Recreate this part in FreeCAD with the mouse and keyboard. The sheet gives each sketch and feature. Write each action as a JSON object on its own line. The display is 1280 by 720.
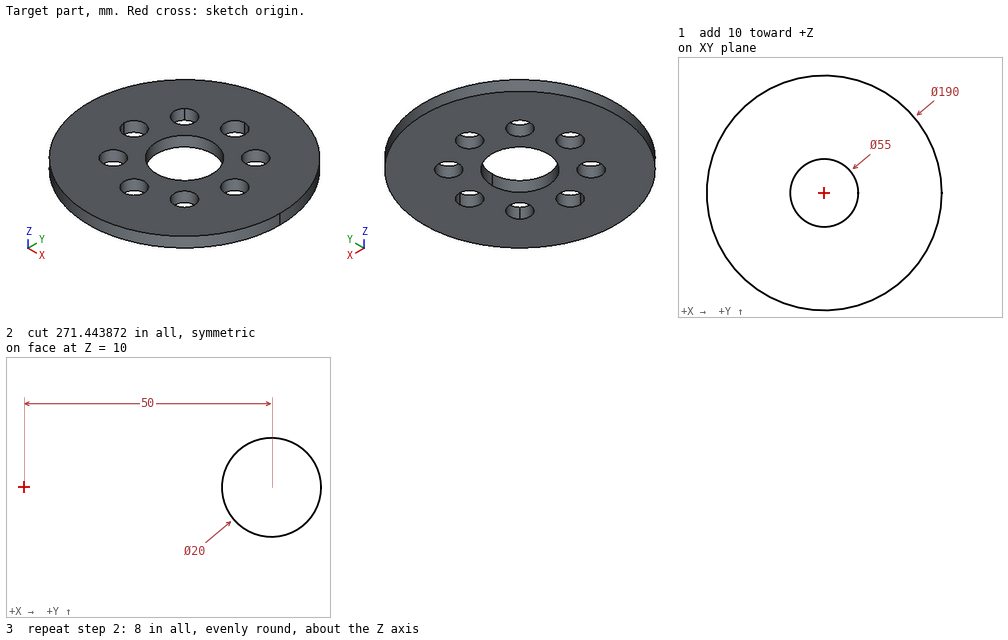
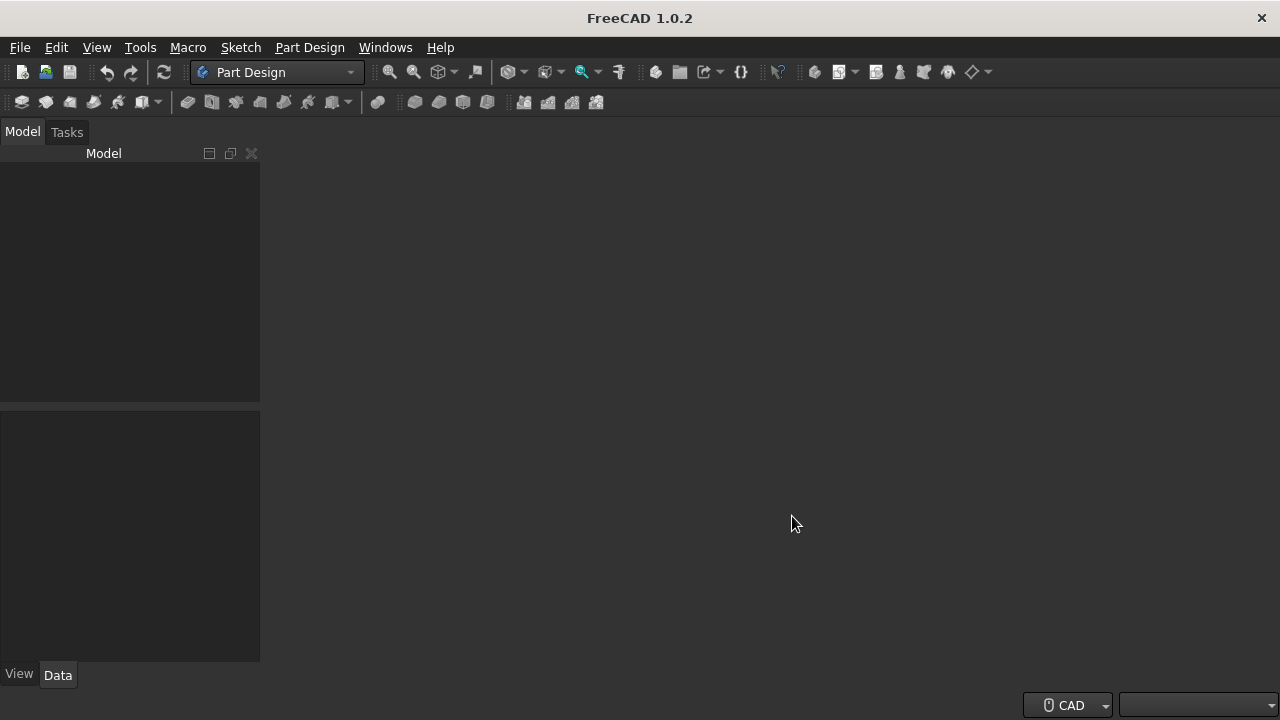
{"action": "left_click", "coordinate": [22, 72]}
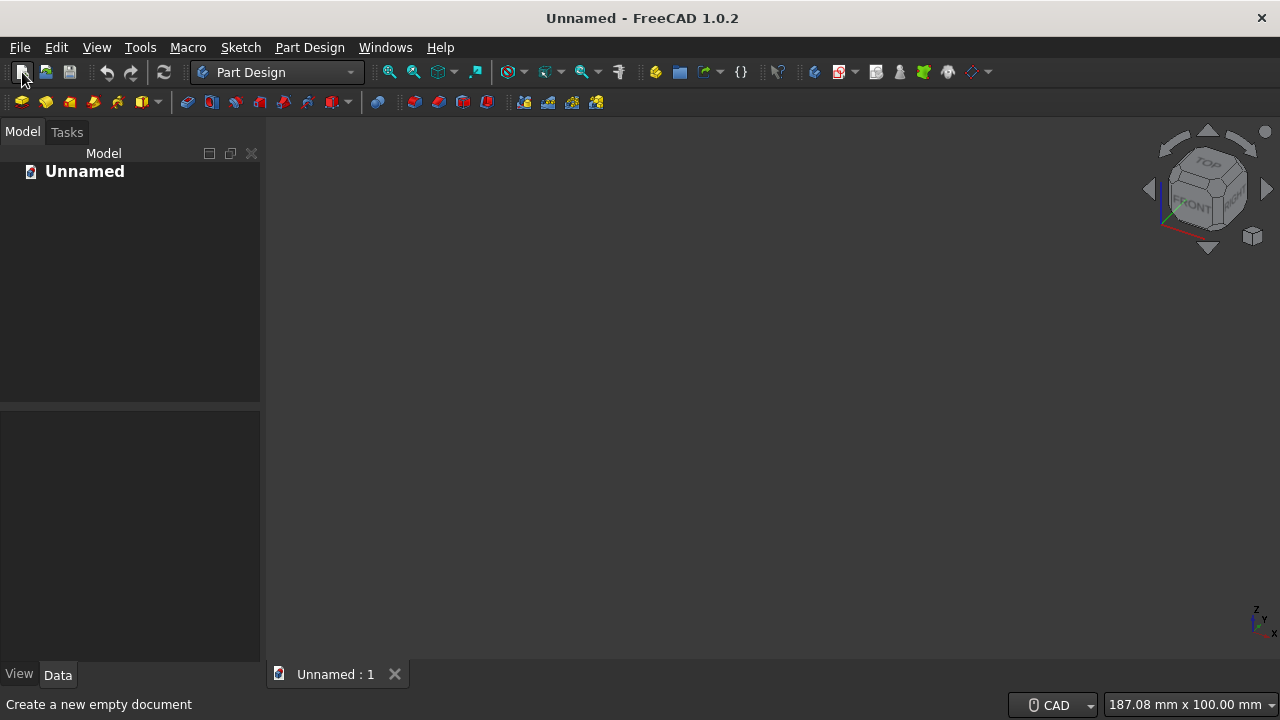
{"action": "left_click", "coordinate": [840, 72]}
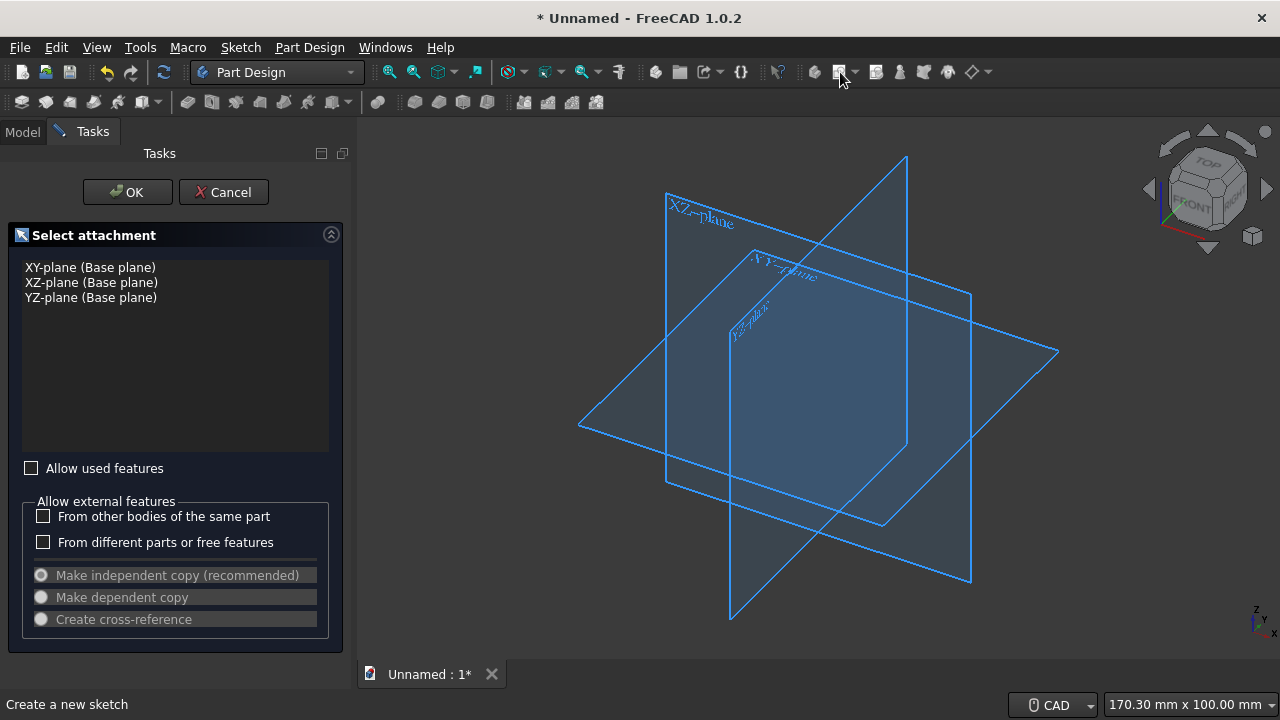
{"action": "left_click", "coordinate": [82, 268]}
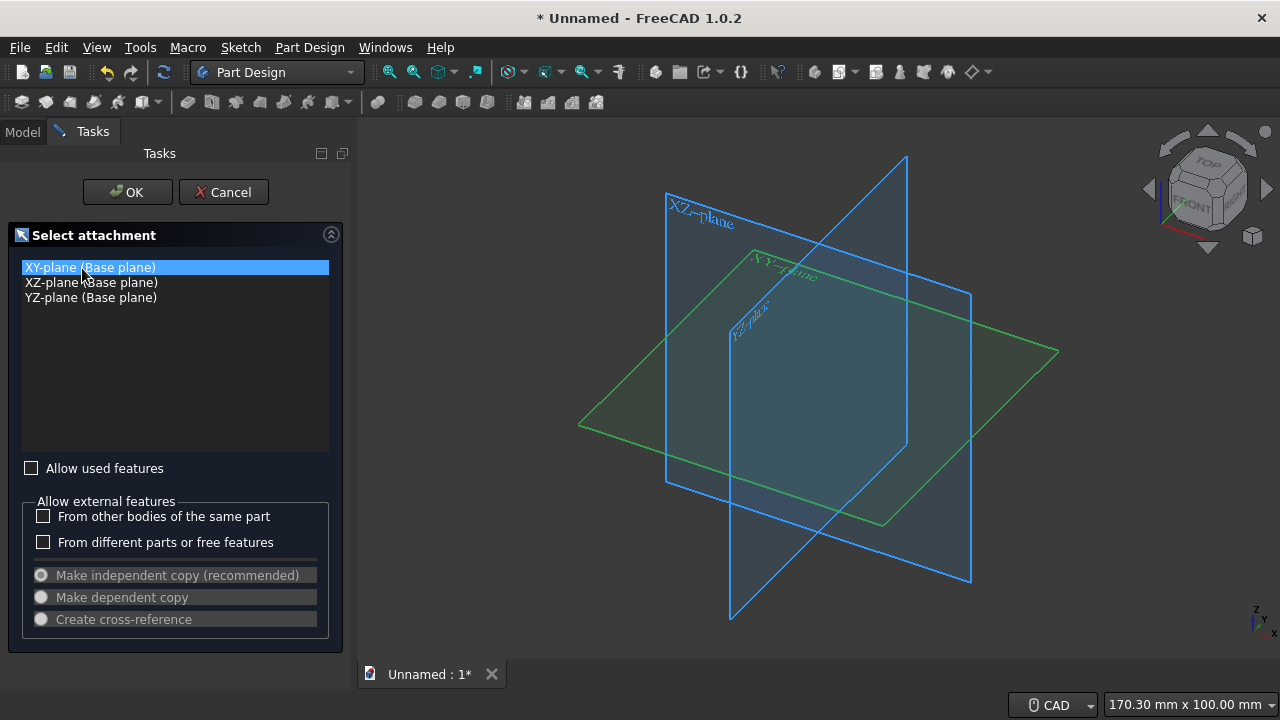
{"action": "left_click", "coordinate": [128, 192]}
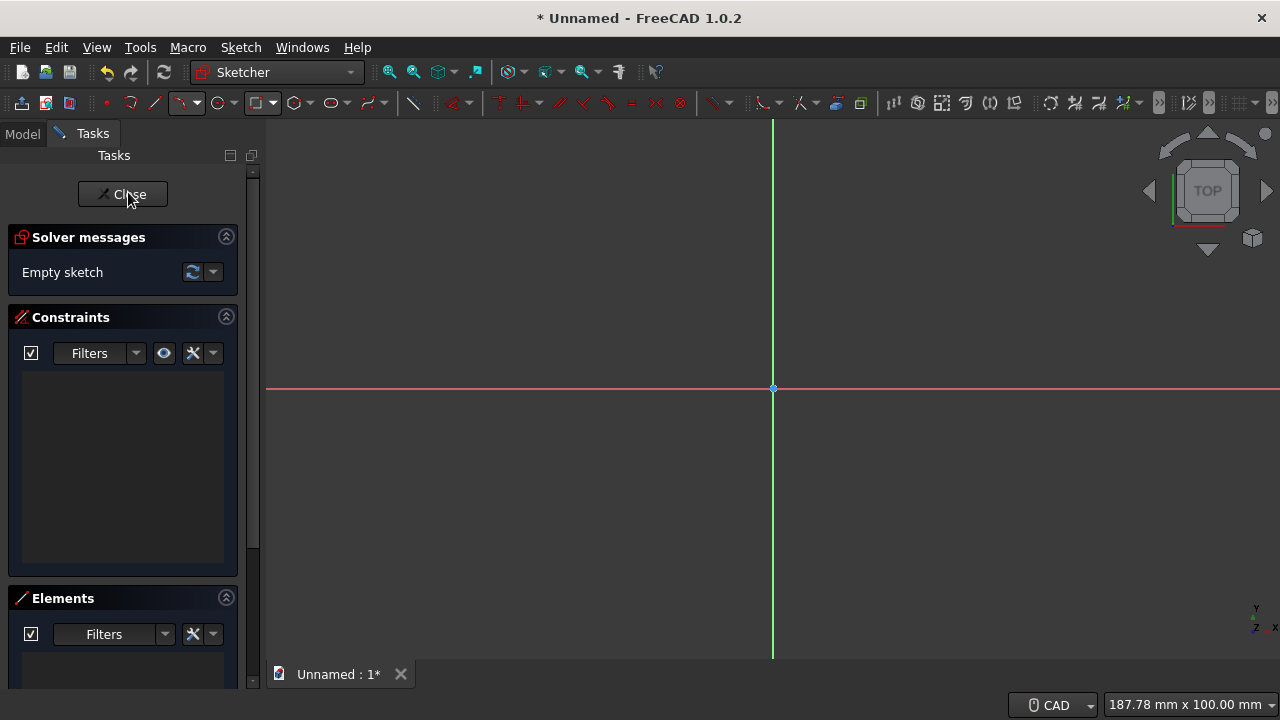
{"action": "scroll", "coordinate": [665, 389], "scroll_direction": "down", "scroll_amount": 5}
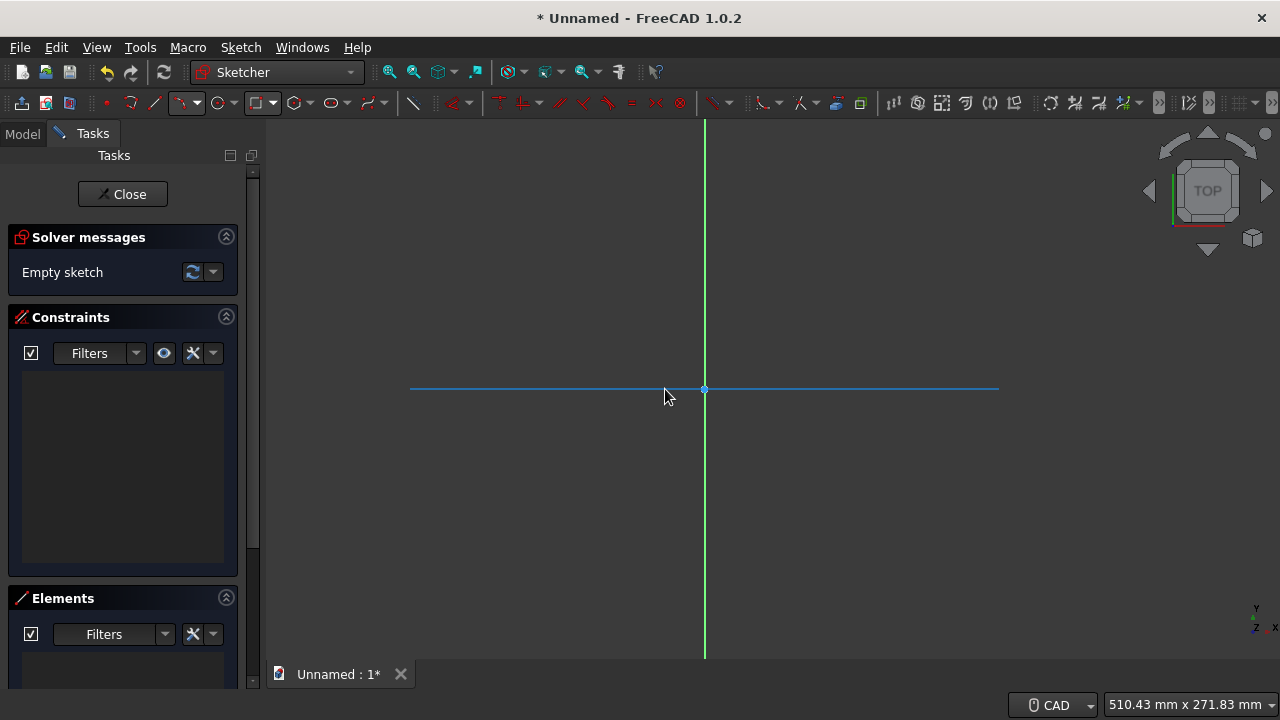
{"action": "left_click", "coordinate": [218, 104]}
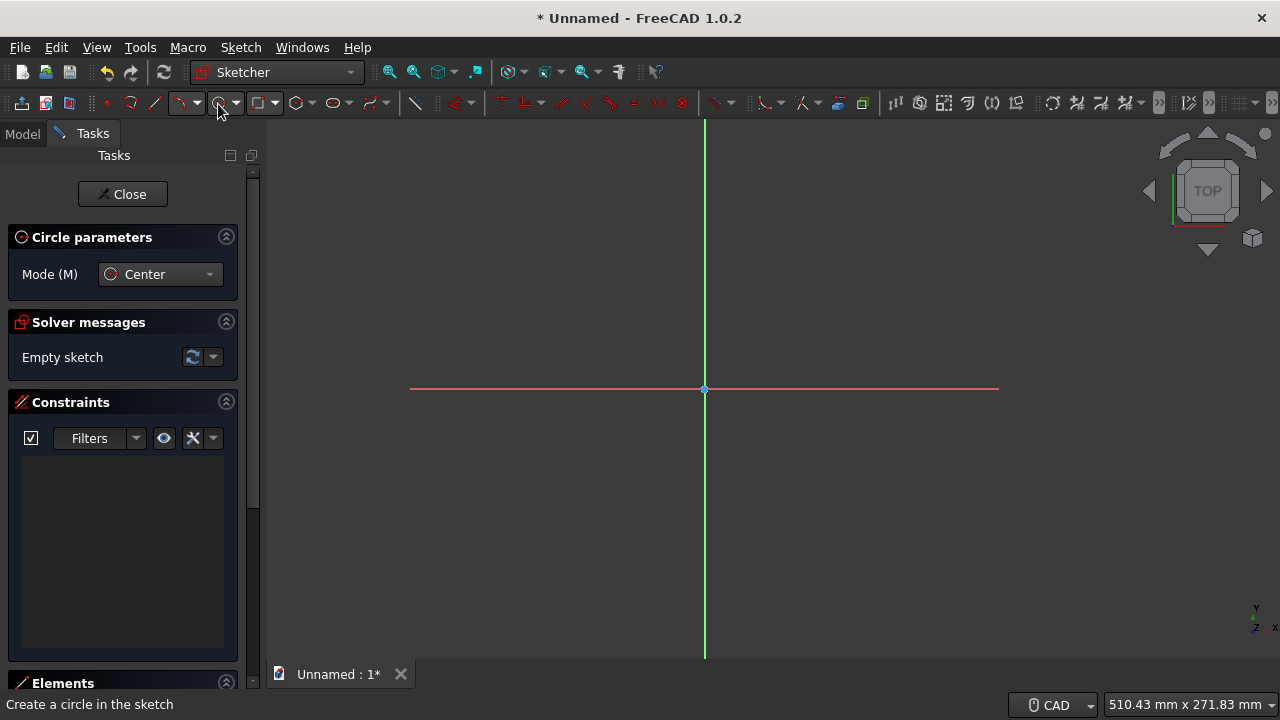
{"action": "left_click", "coordinate": [705, 389]}
{"action": "mouse_move", "coordinate": [838, 256]}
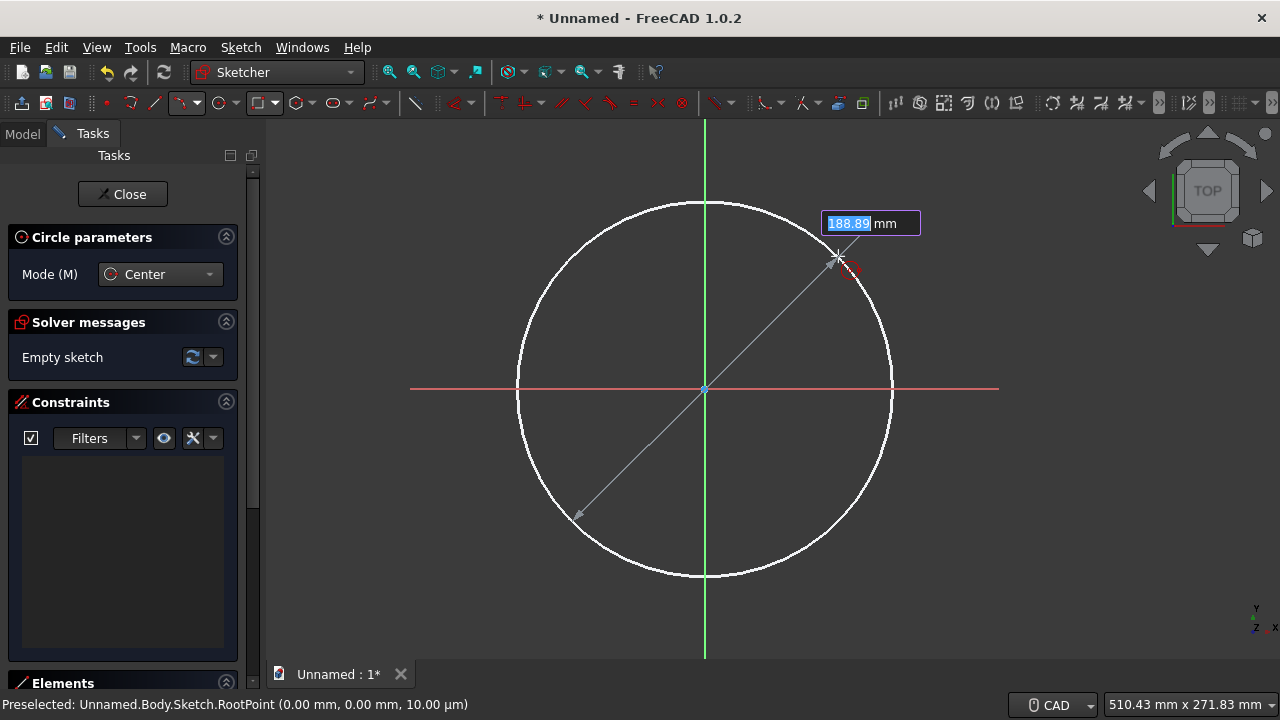
{"action": "type", "text": "190"}
{"action": "key", "text": "Return"}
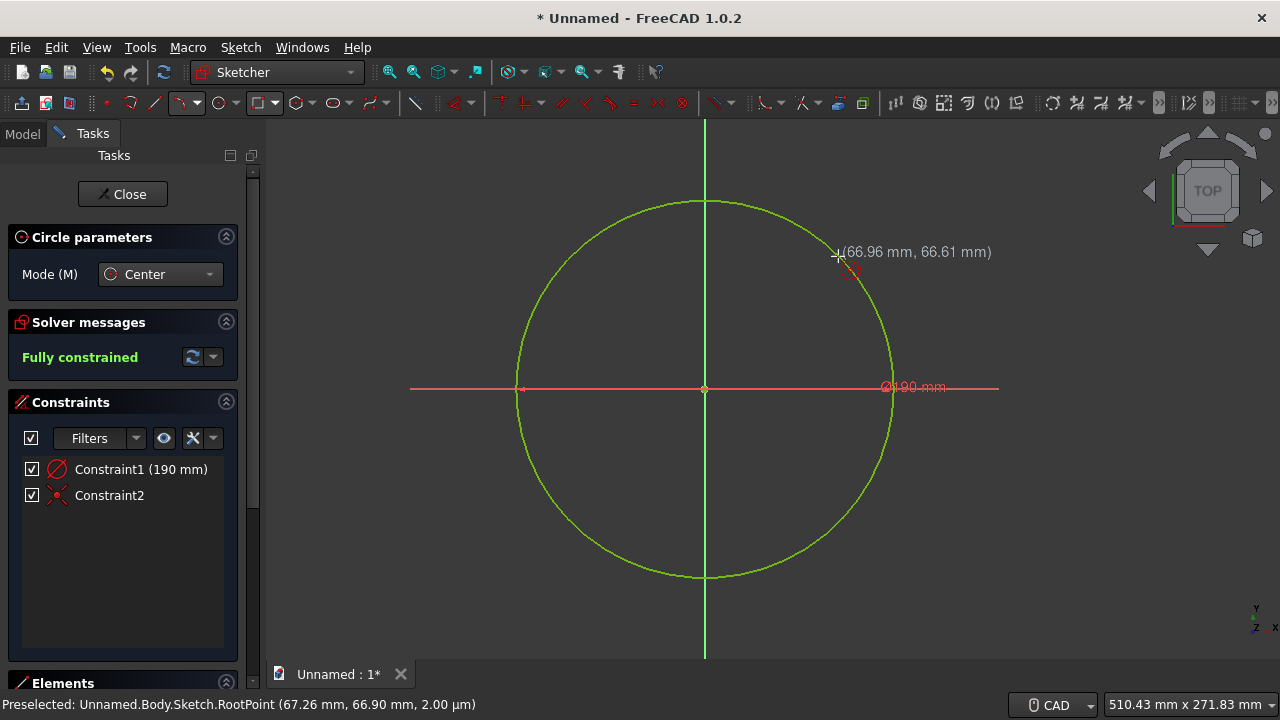
{"action": "left_click", "coordinate": [705, 389]}
{"action": "mouse_move", "coordinate": [744, 351]}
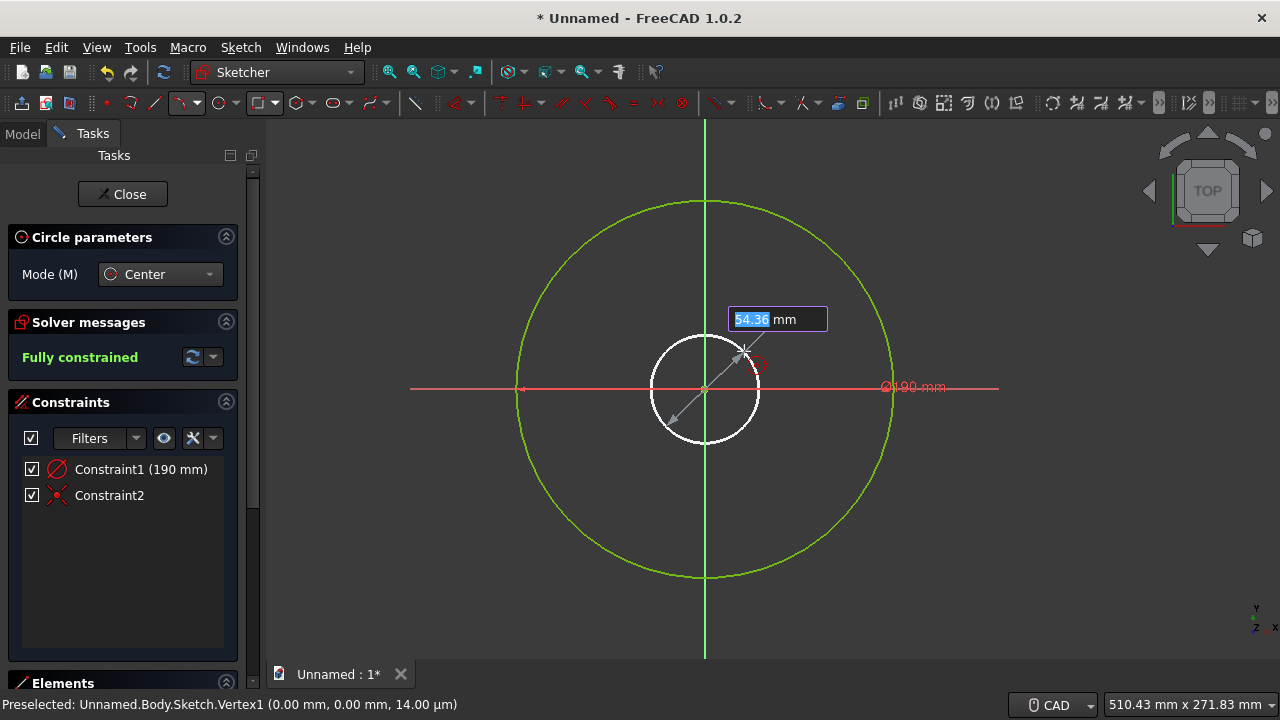
{"action": "type", "text": "55"}
{"action": "key", "text": "Return"}
{"action": "key", "text": "Escape"}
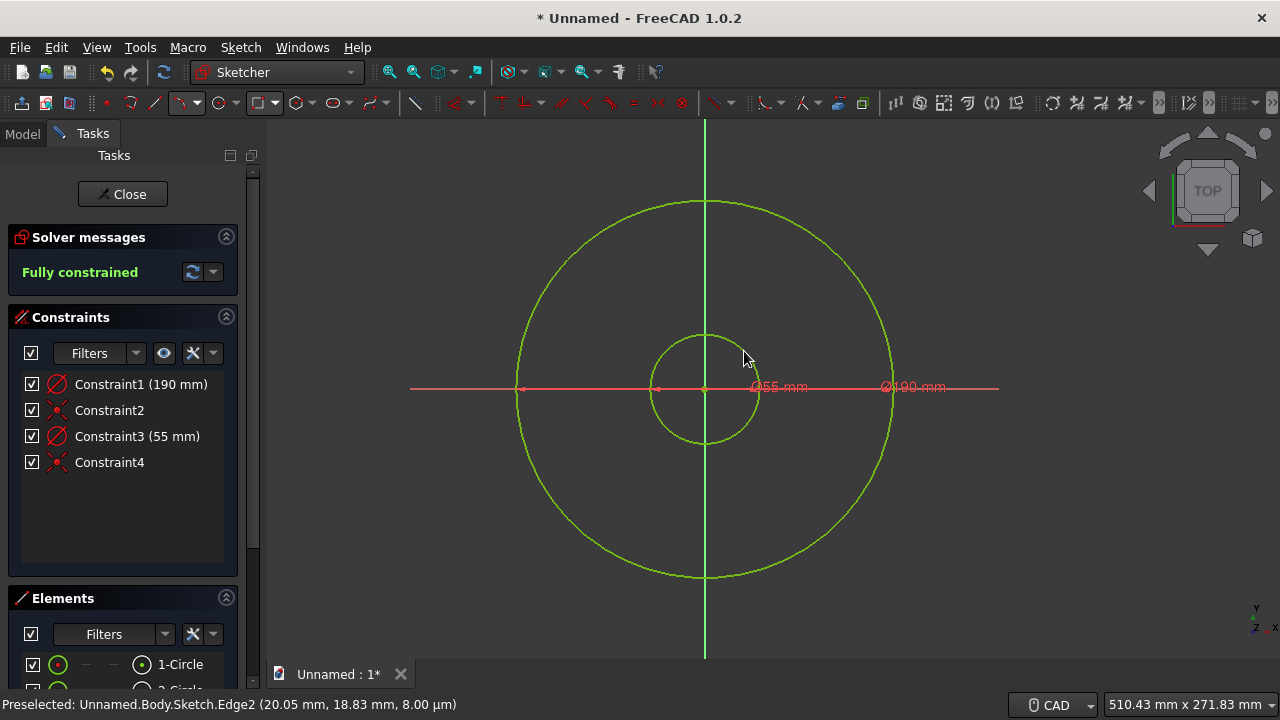
{"action": "left_click", "coordinate": [123, 194]}